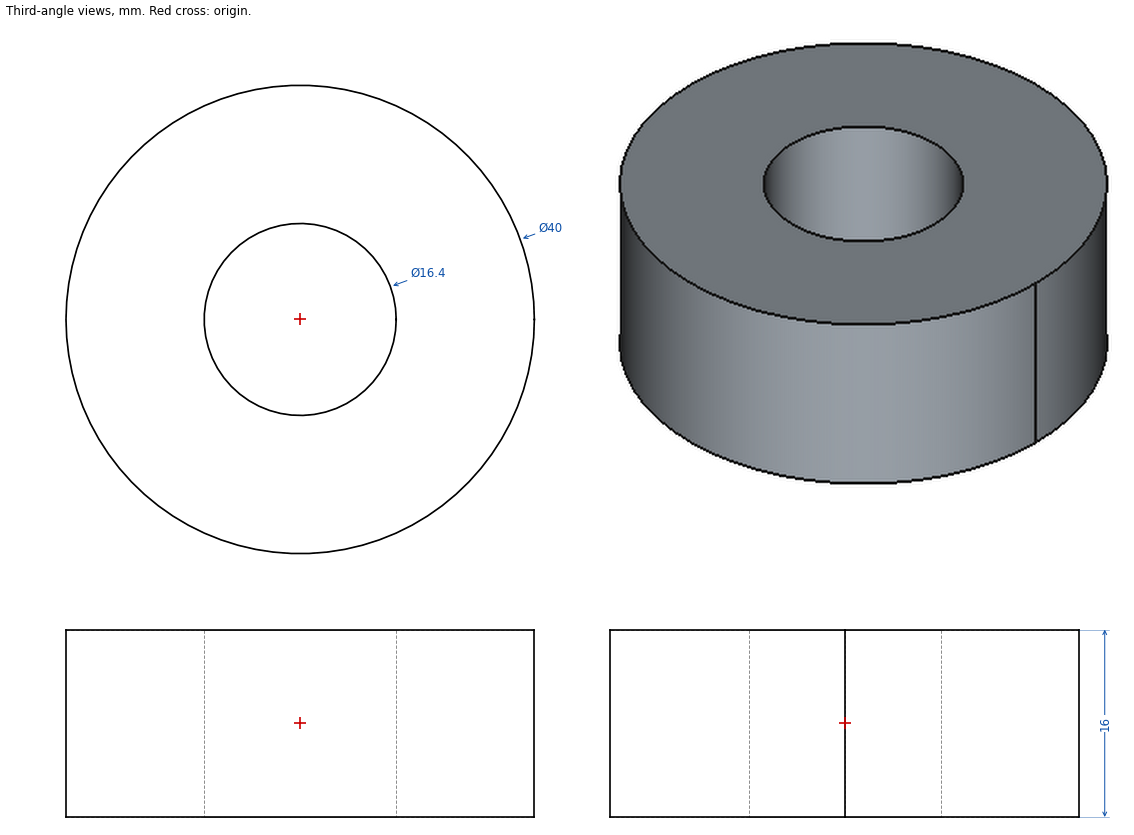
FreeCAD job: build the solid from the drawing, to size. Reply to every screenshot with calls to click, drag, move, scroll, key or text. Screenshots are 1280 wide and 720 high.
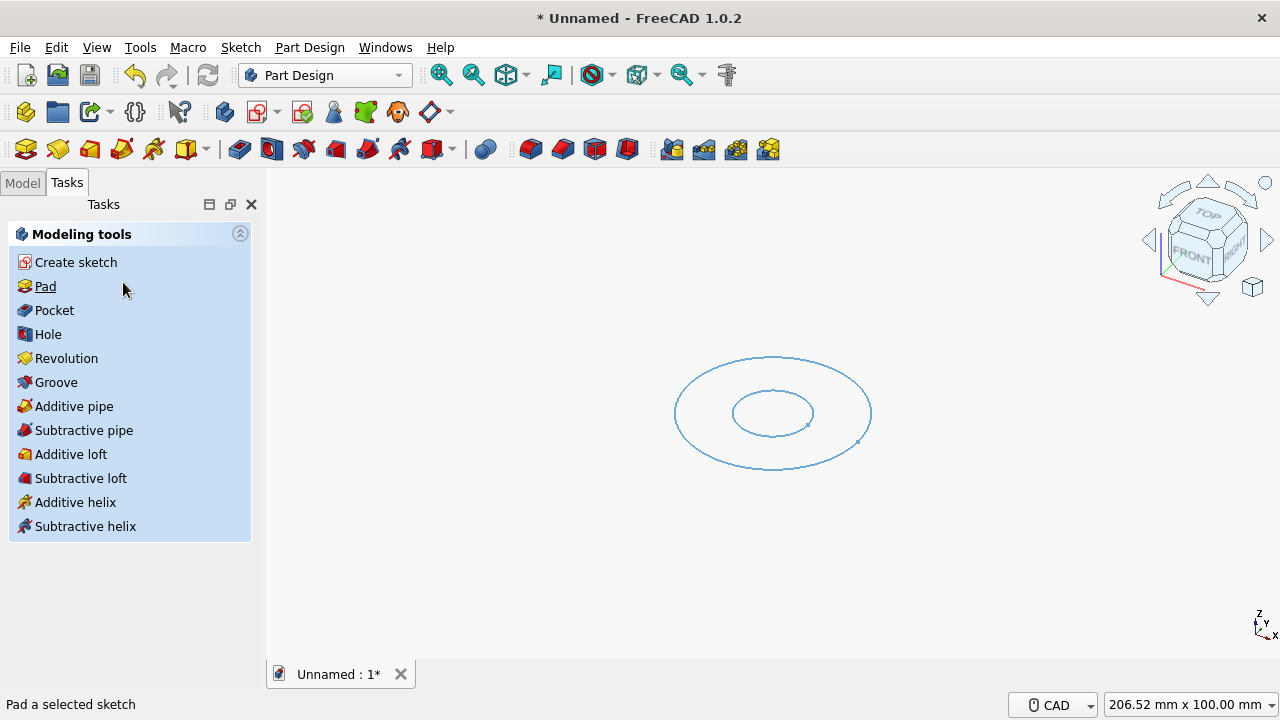
click(26, 150)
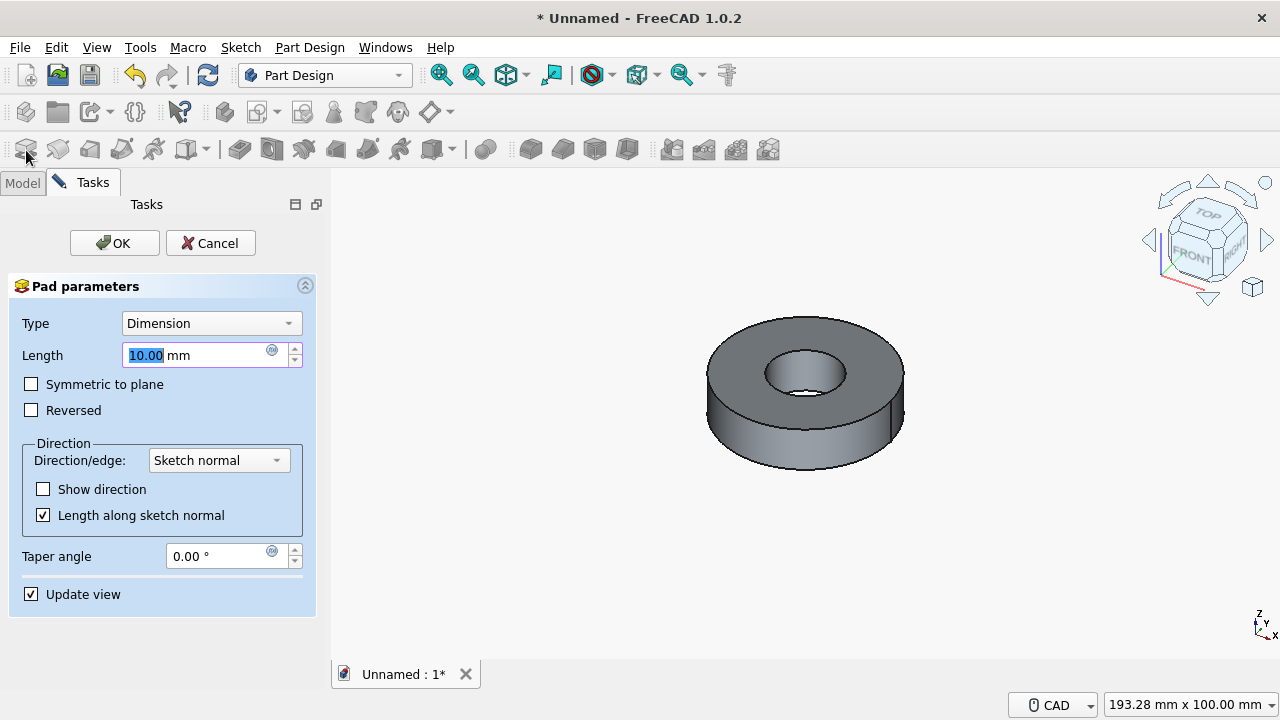
text(16)
key(Tab)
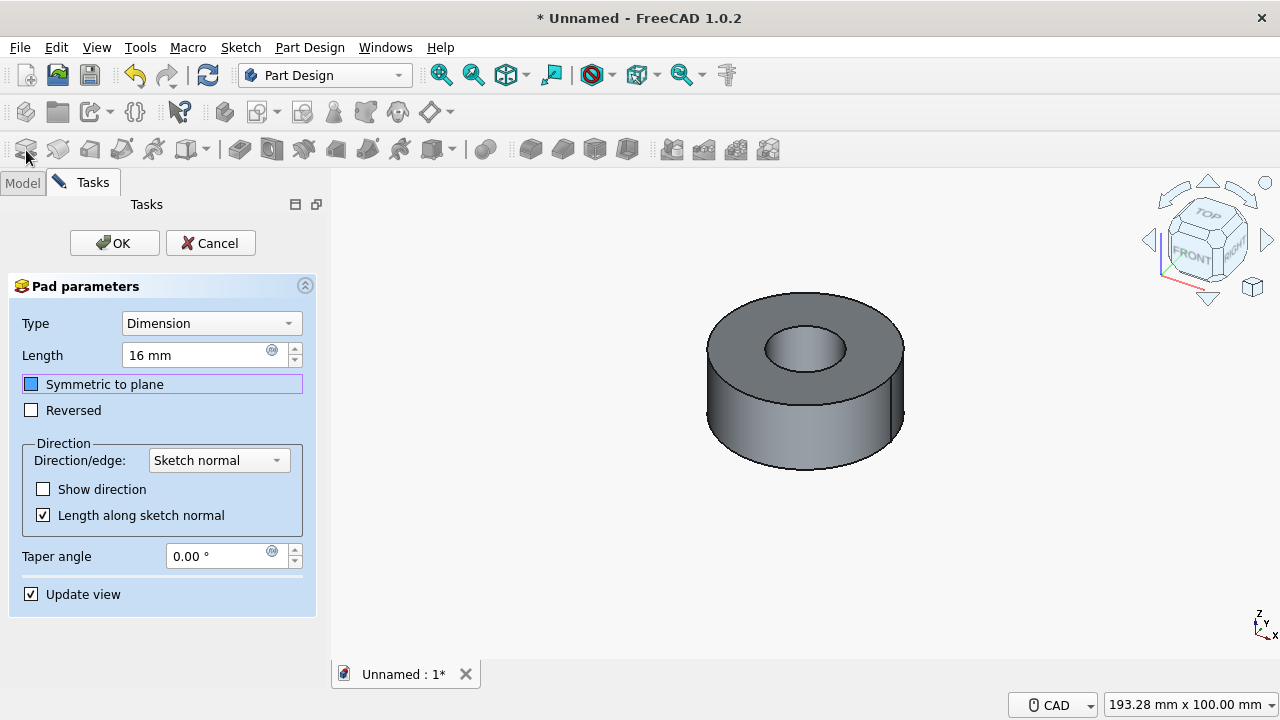
click(30, 384)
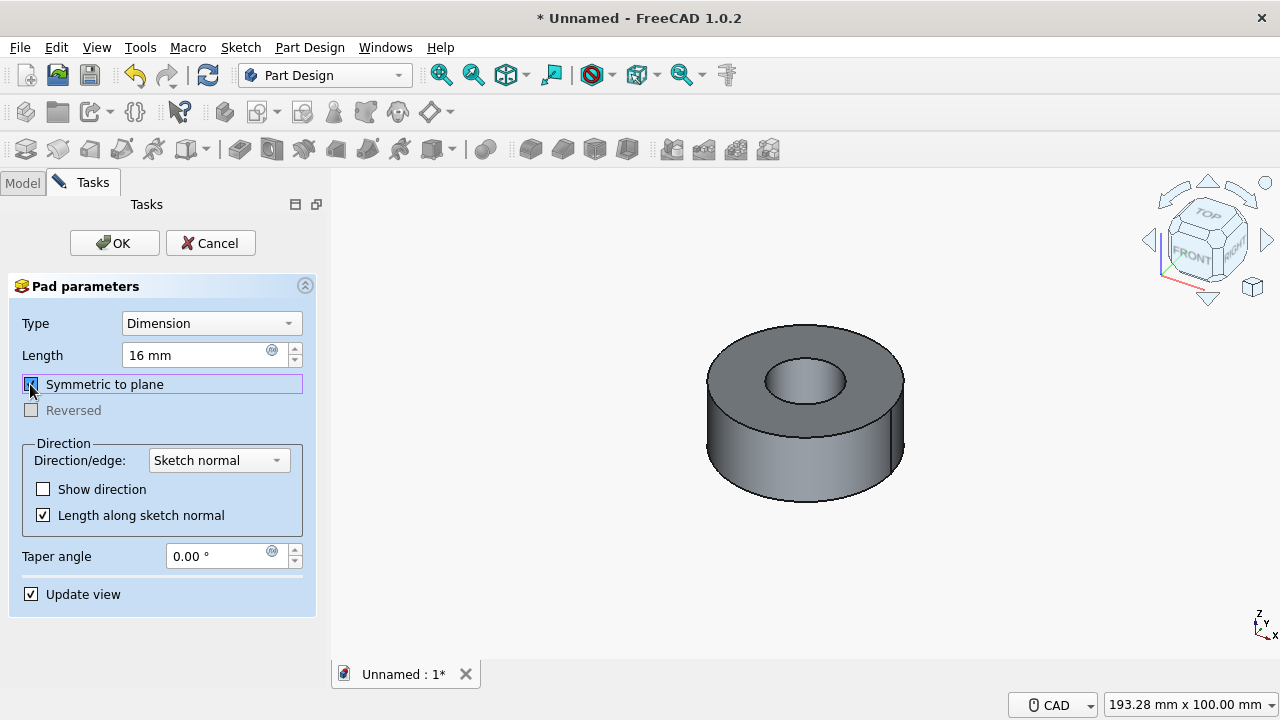
click(115, 243)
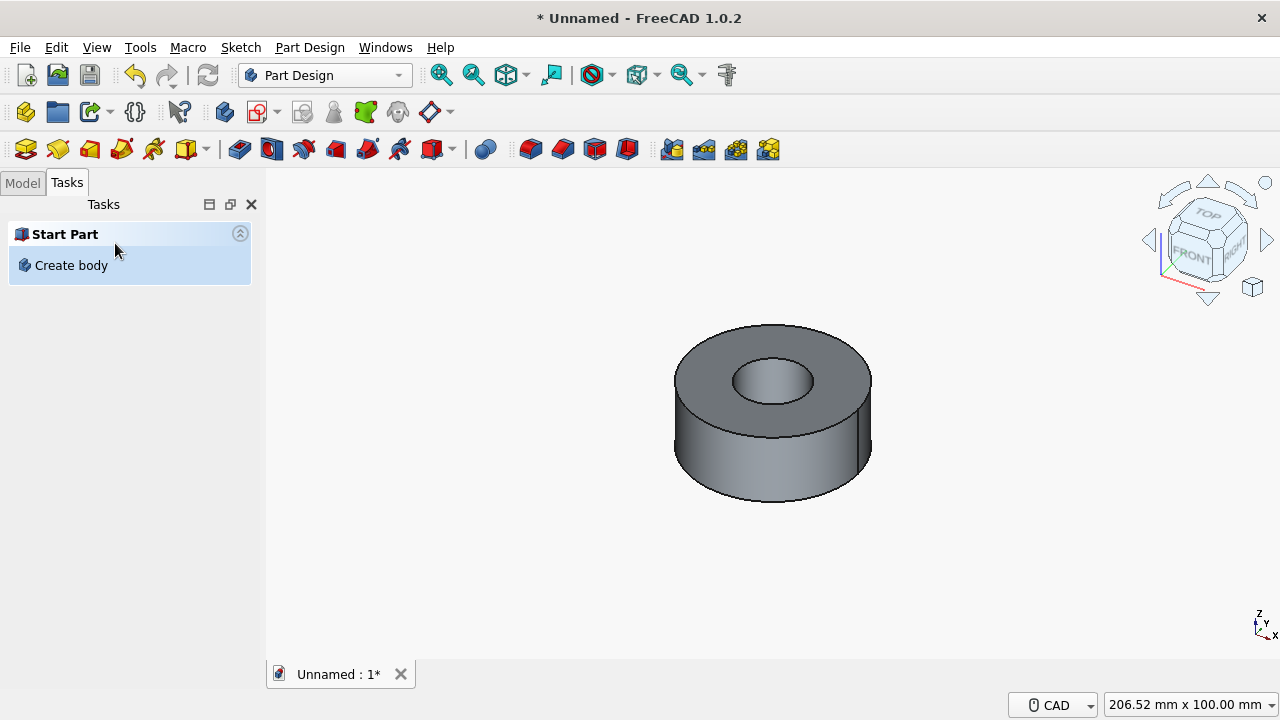
key(0)